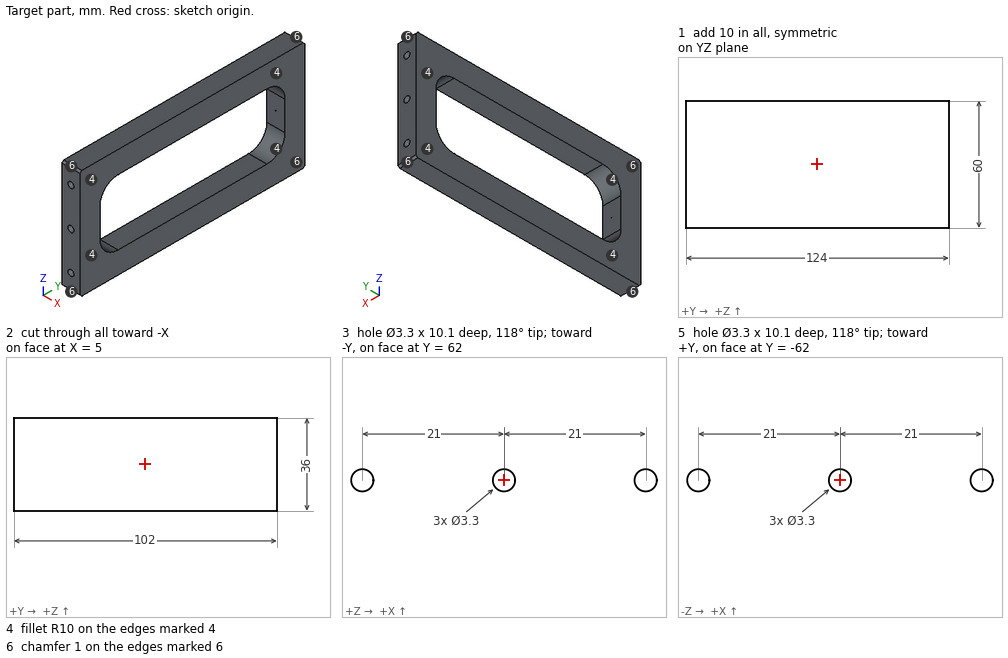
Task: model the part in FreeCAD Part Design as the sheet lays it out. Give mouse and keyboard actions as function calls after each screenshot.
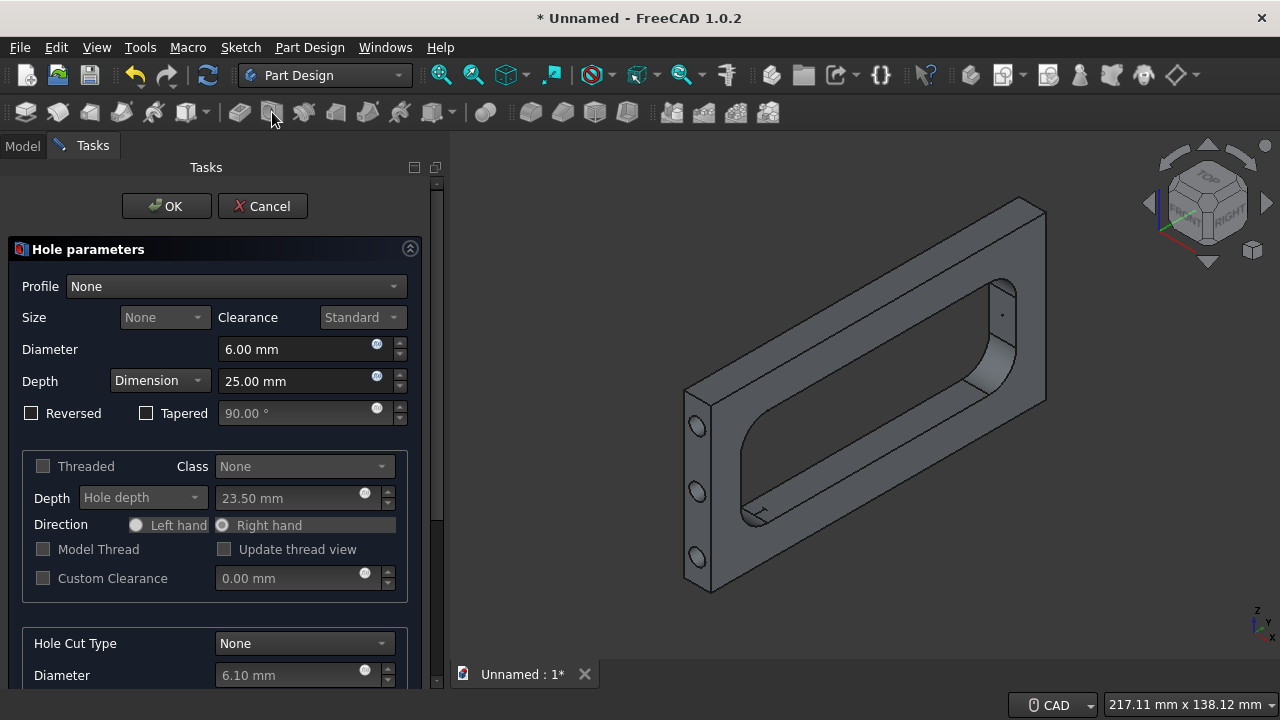
triple_click(305, 349)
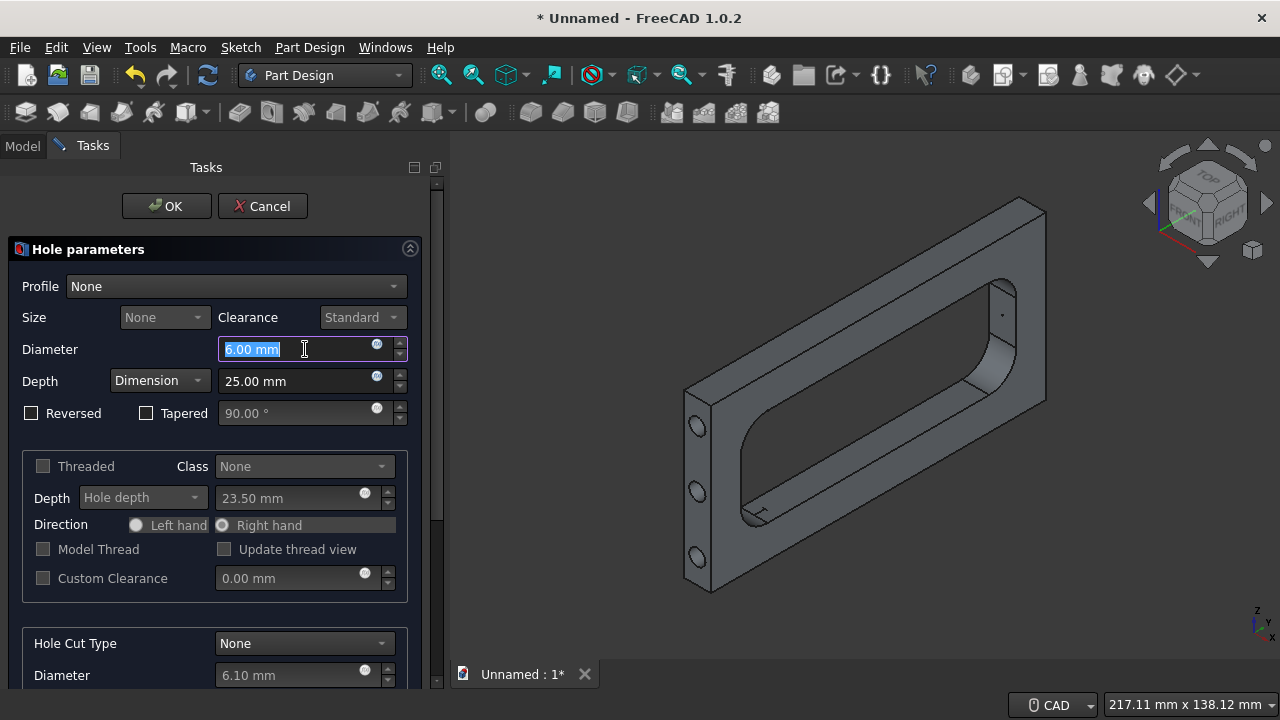
text(3.3)
key(Tab)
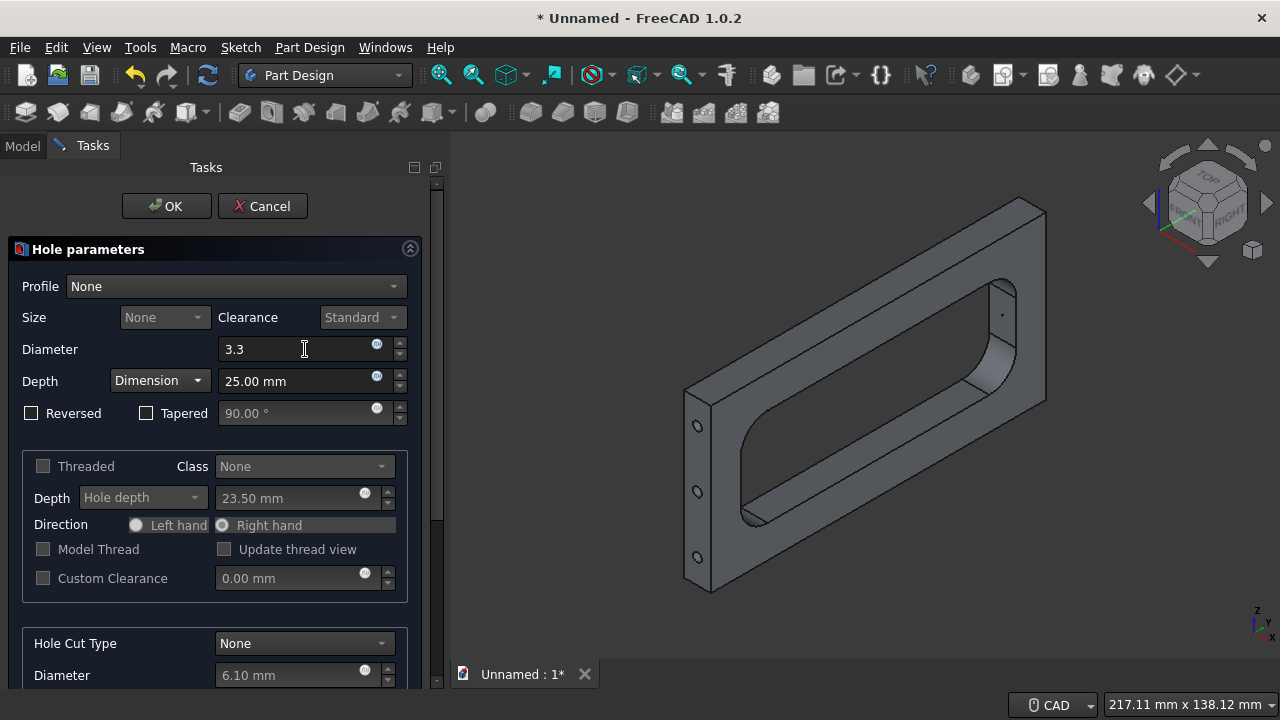
triple_click(305, 381)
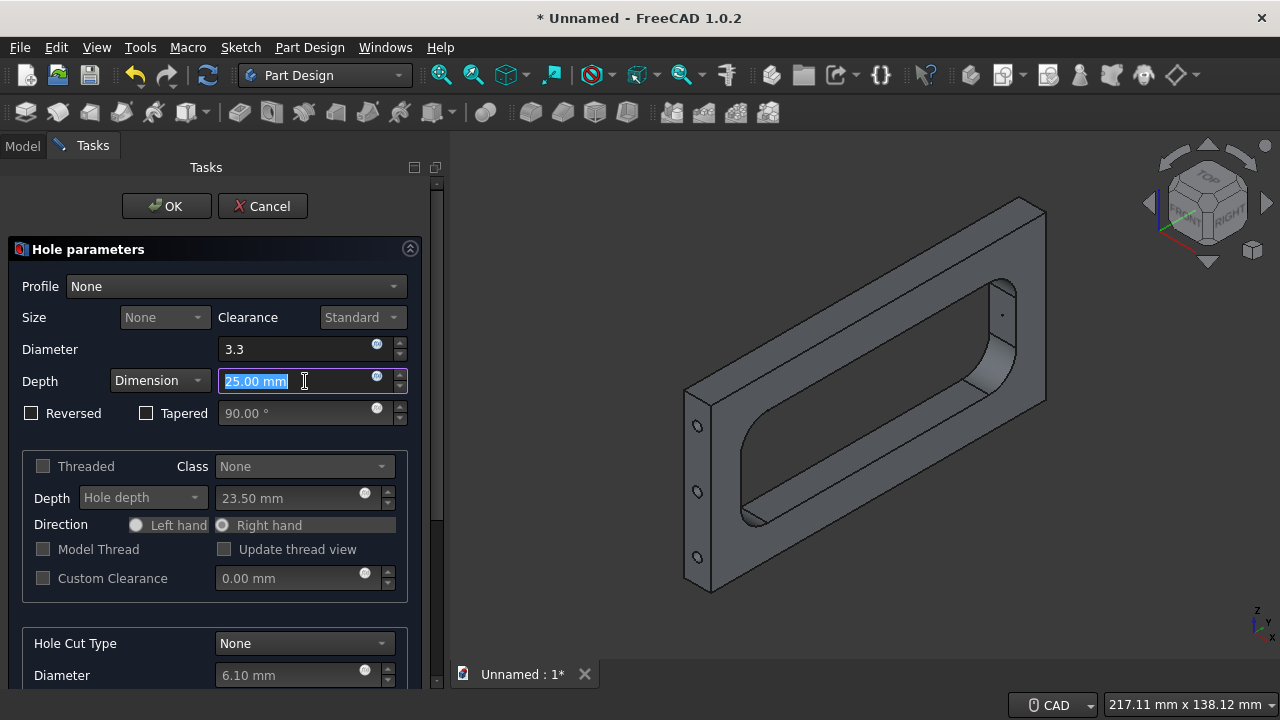
text(10.1)
key(Tab)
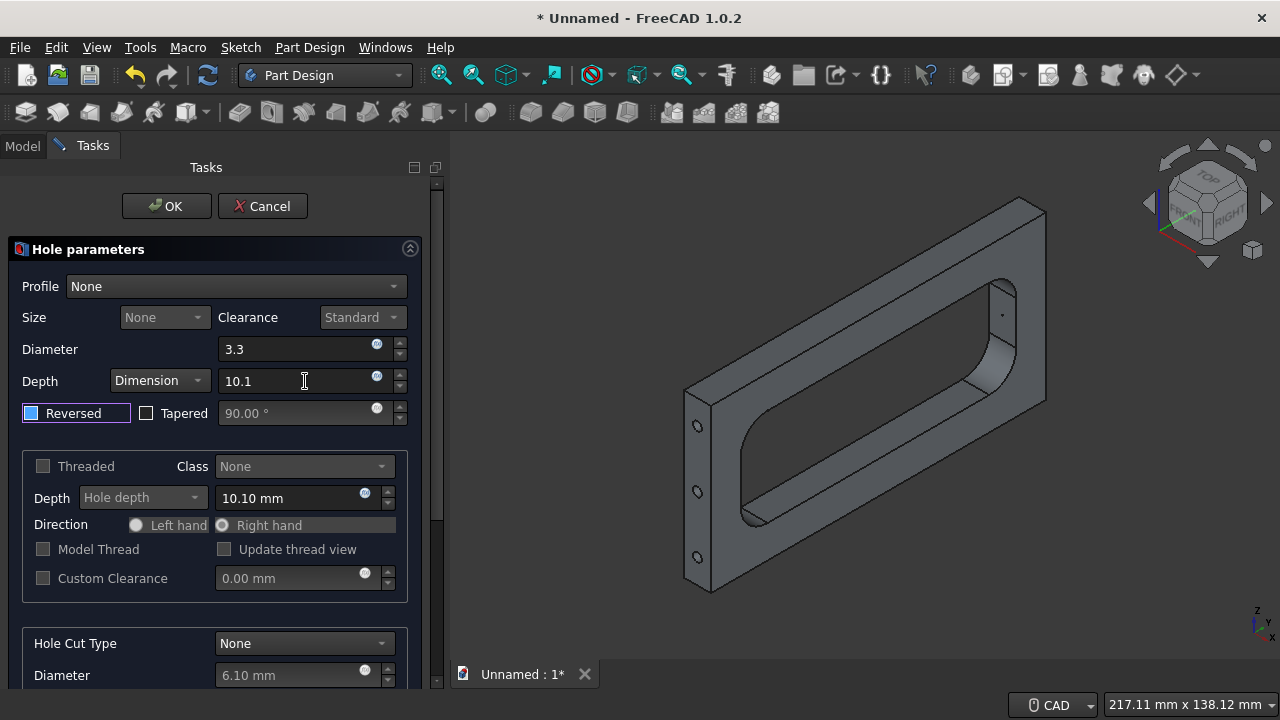
click(167, 206)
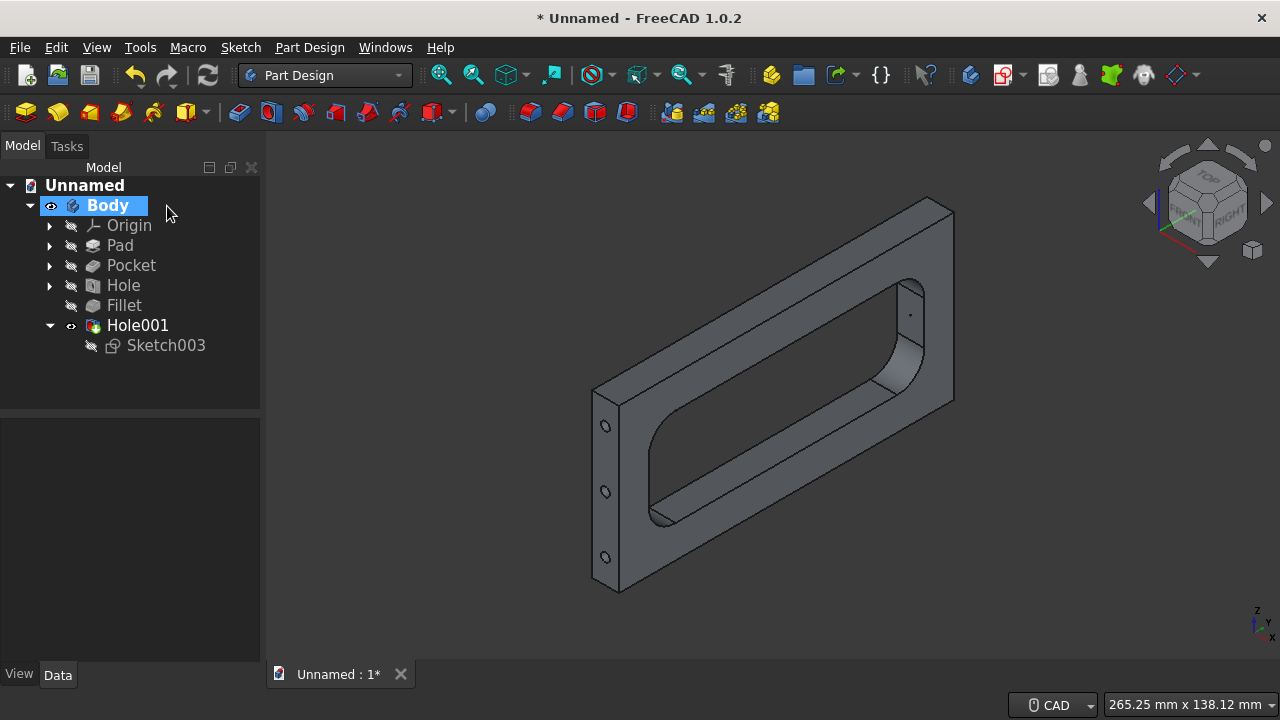
click(605, 397)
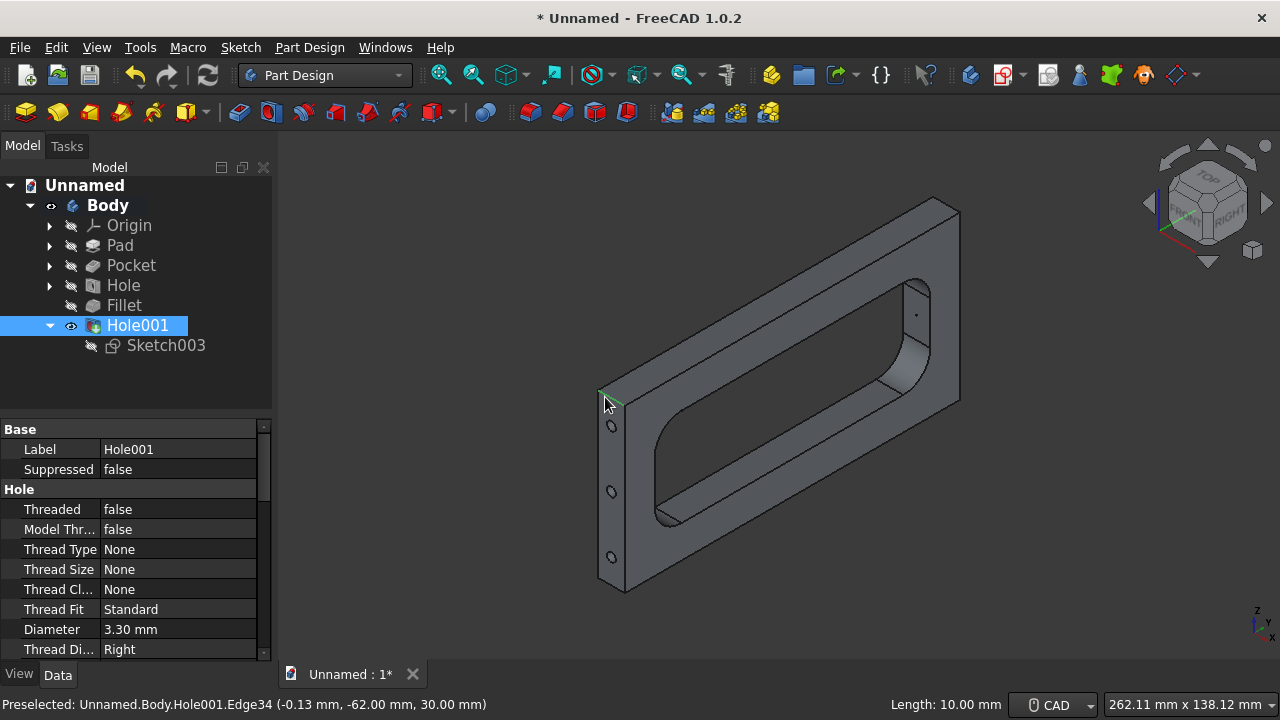
key(2)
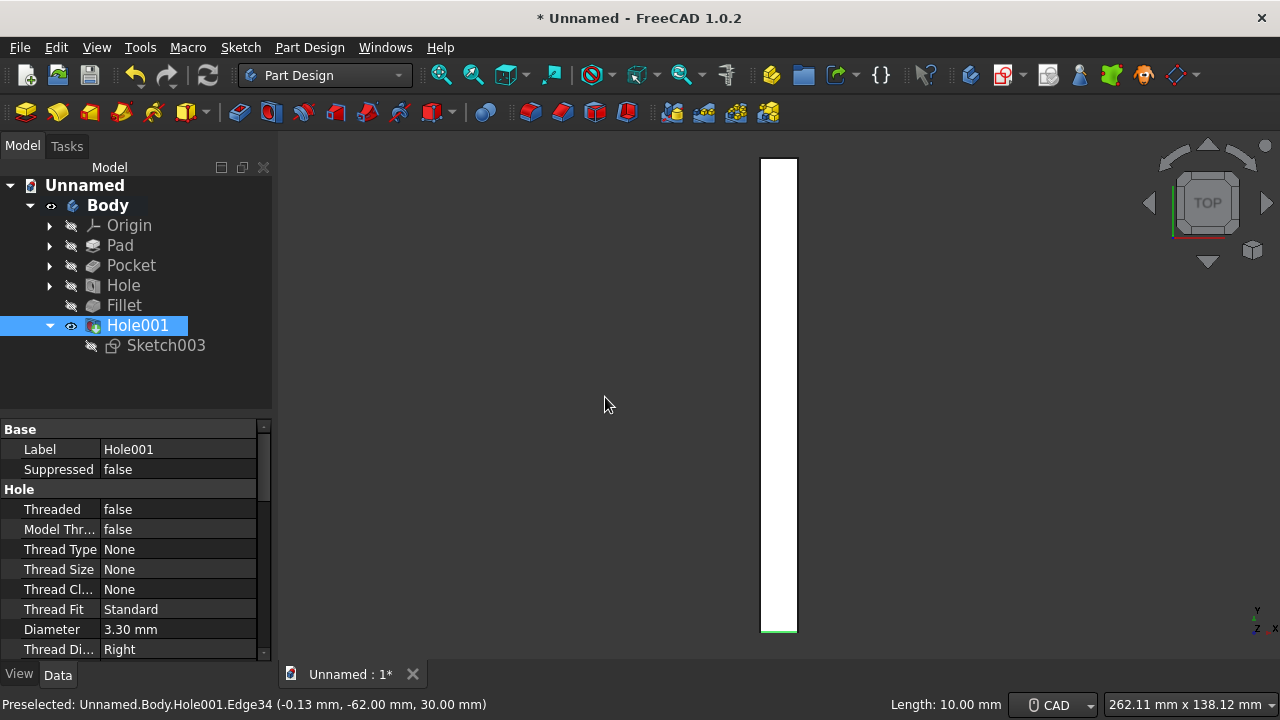
key(0)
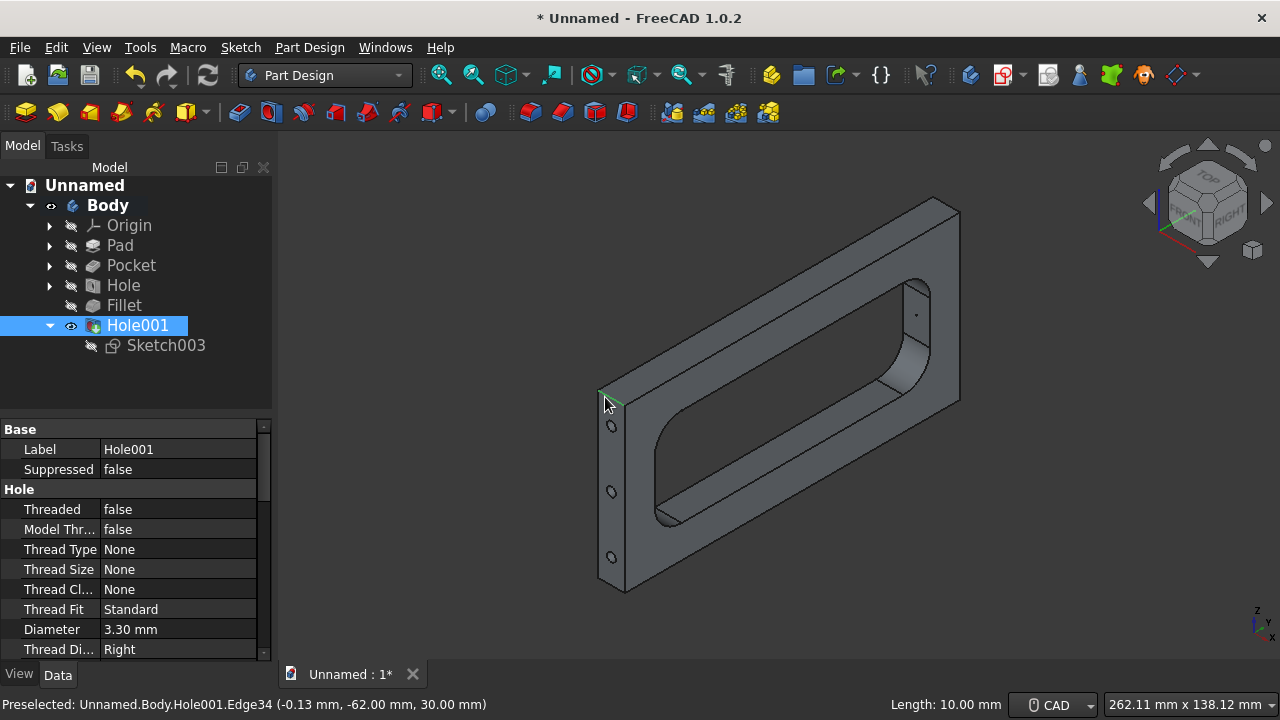
key(1)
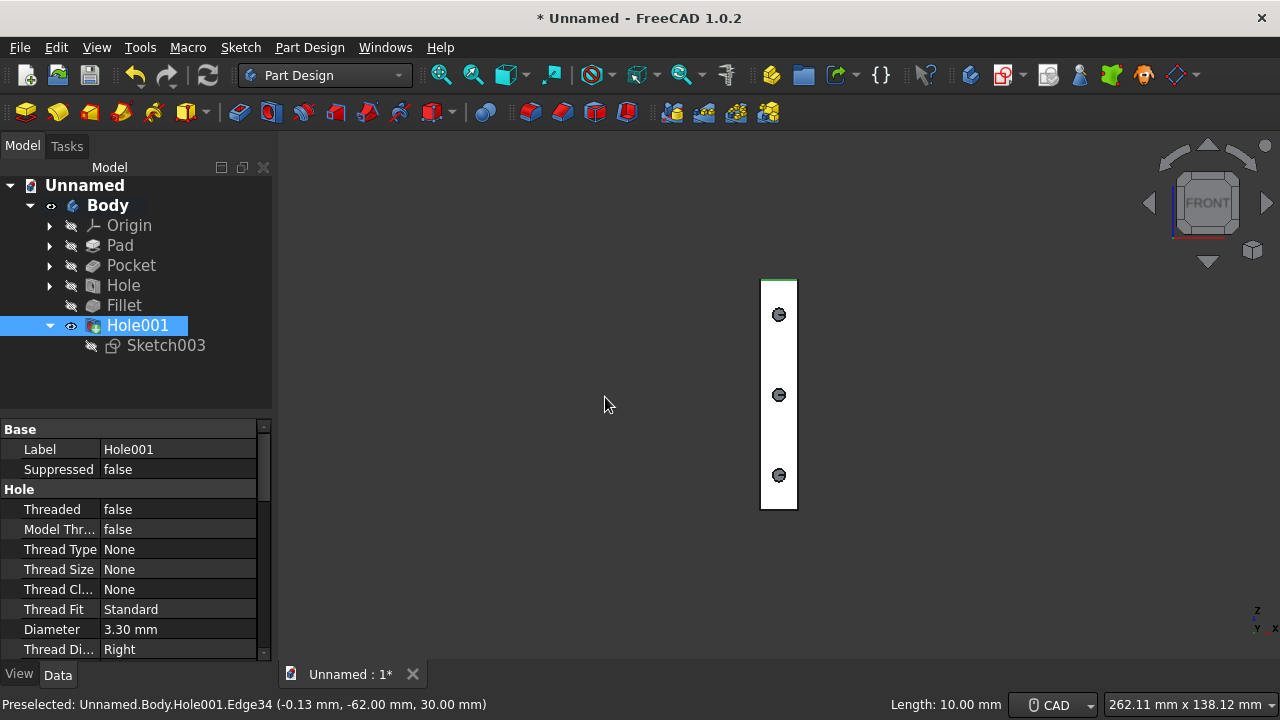
click(442, 76)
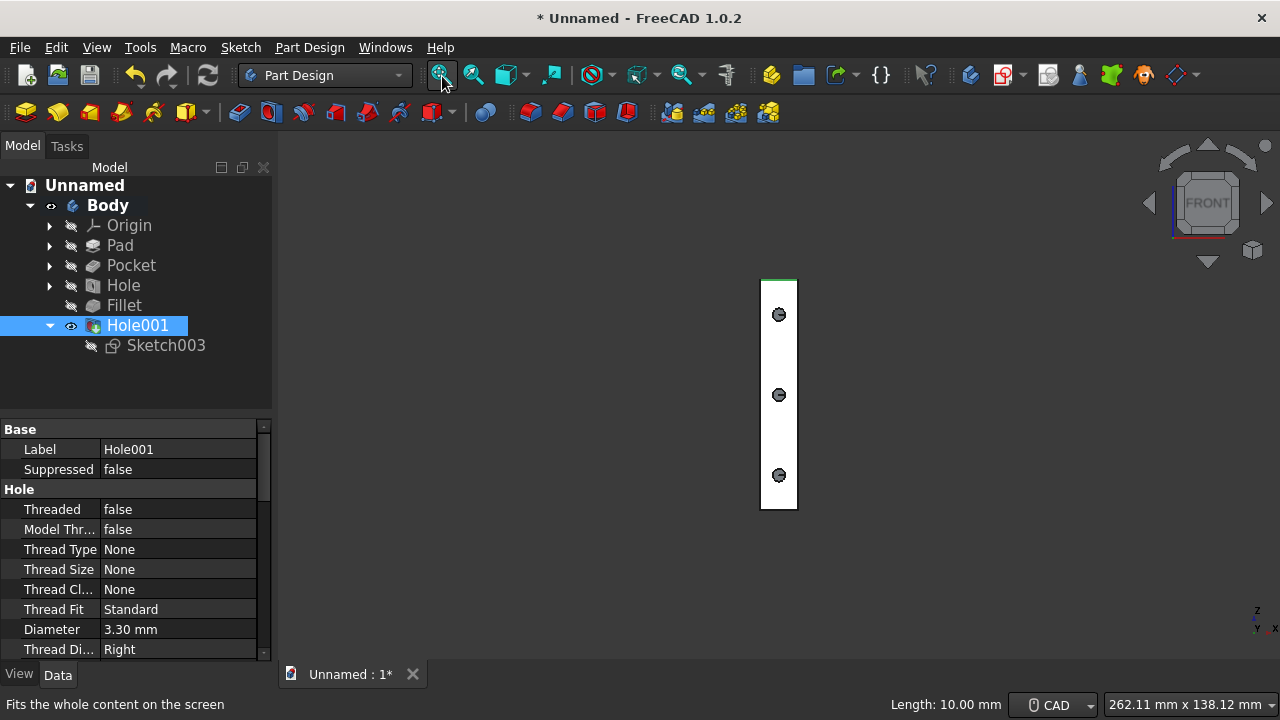
click(779, 509, ctrl)